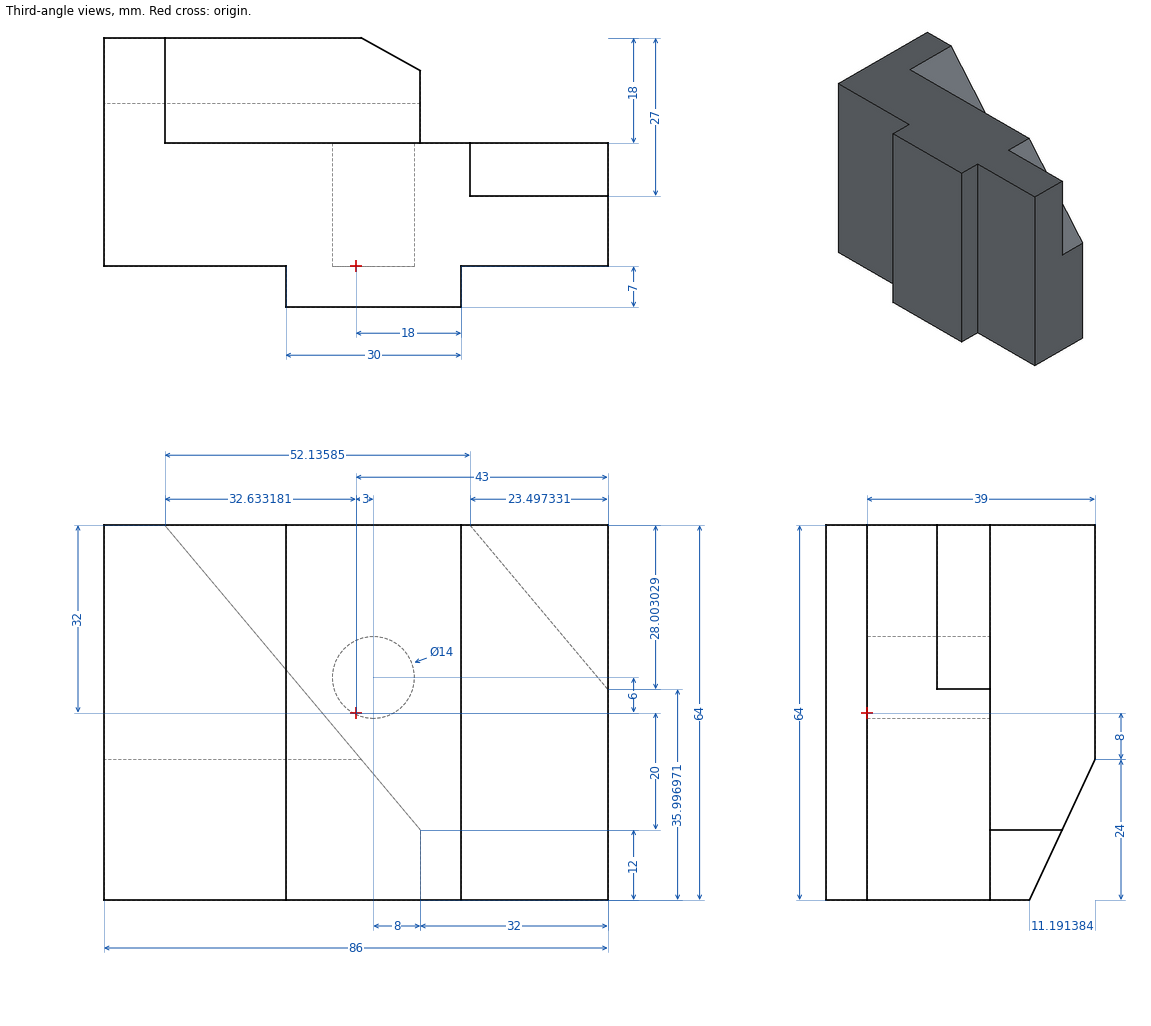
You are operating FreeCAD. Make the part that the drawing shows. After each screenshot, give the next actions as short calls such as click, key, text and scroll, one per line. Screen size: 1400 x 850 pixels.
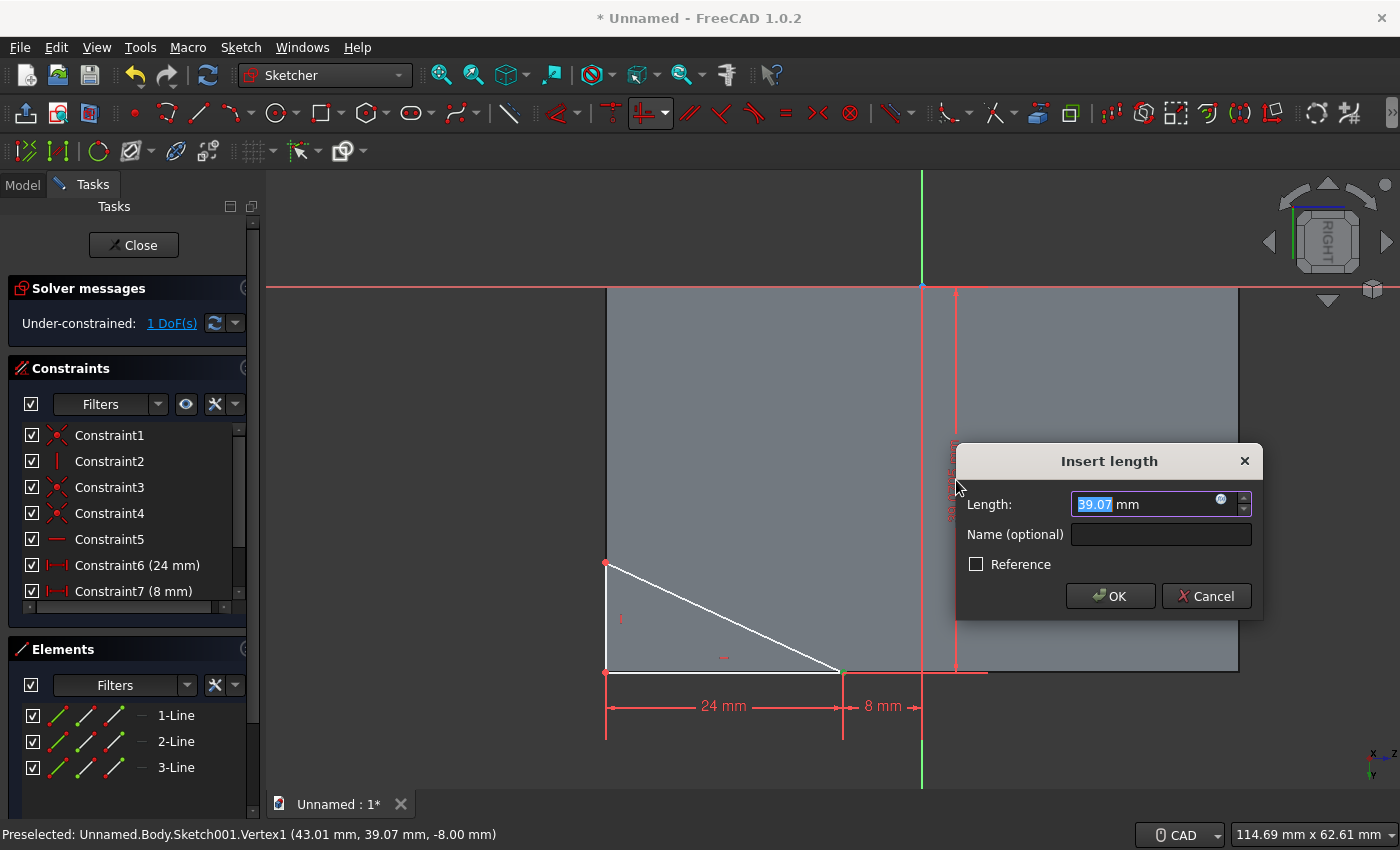
text(39)
key(Return)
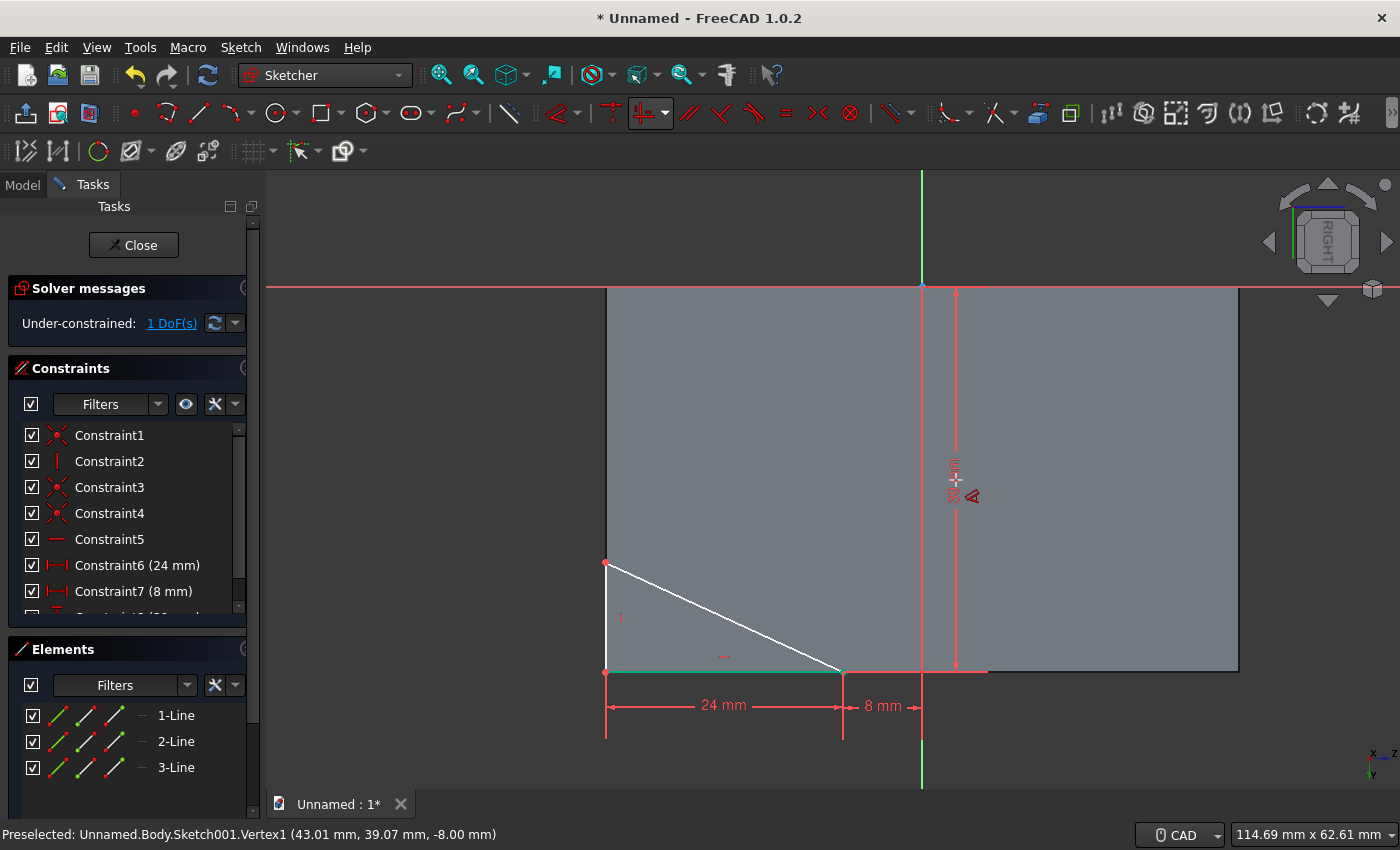
click(606, 596)
click(572, 618)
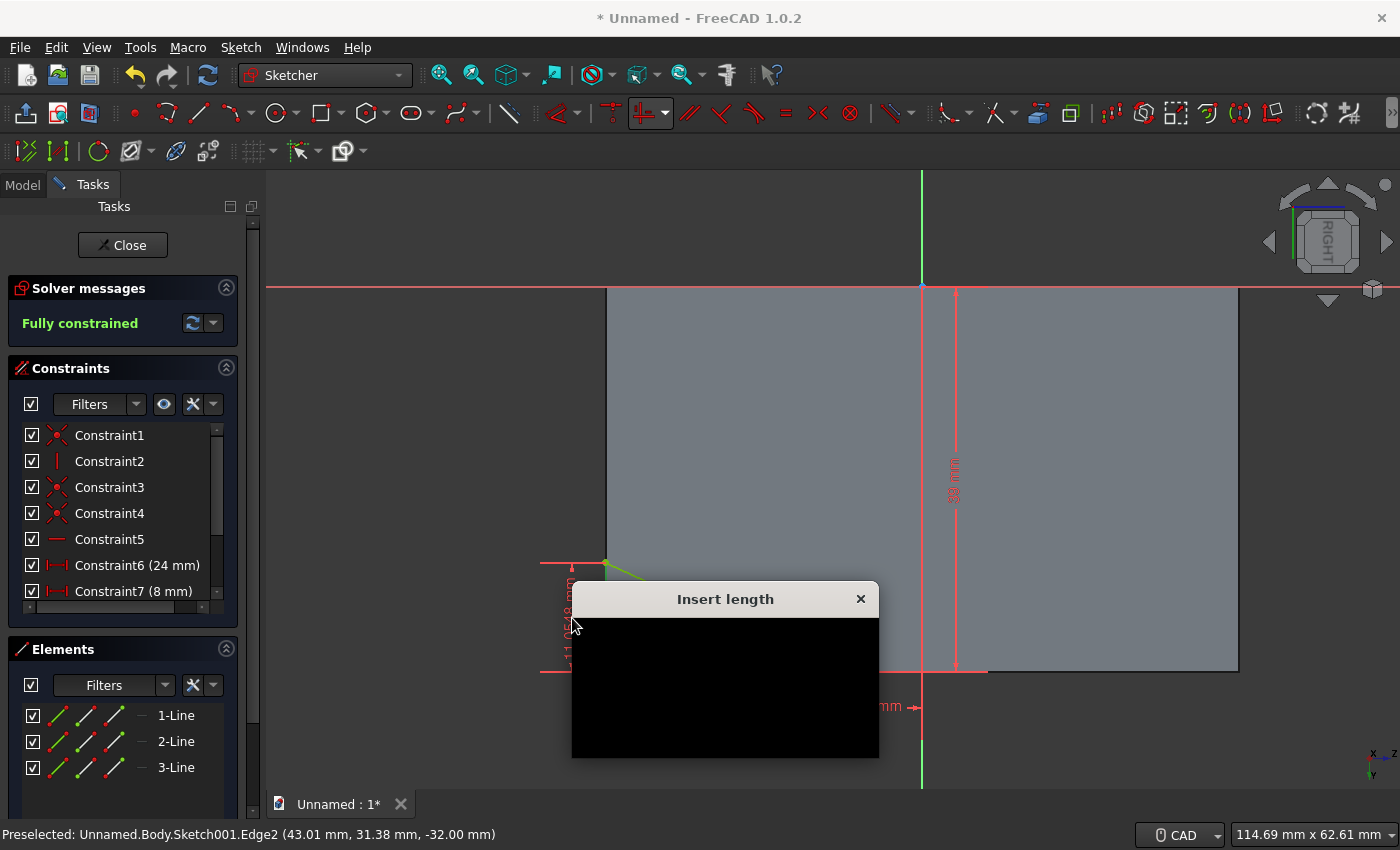
text(11.191384)
key(Return)
key(Escape)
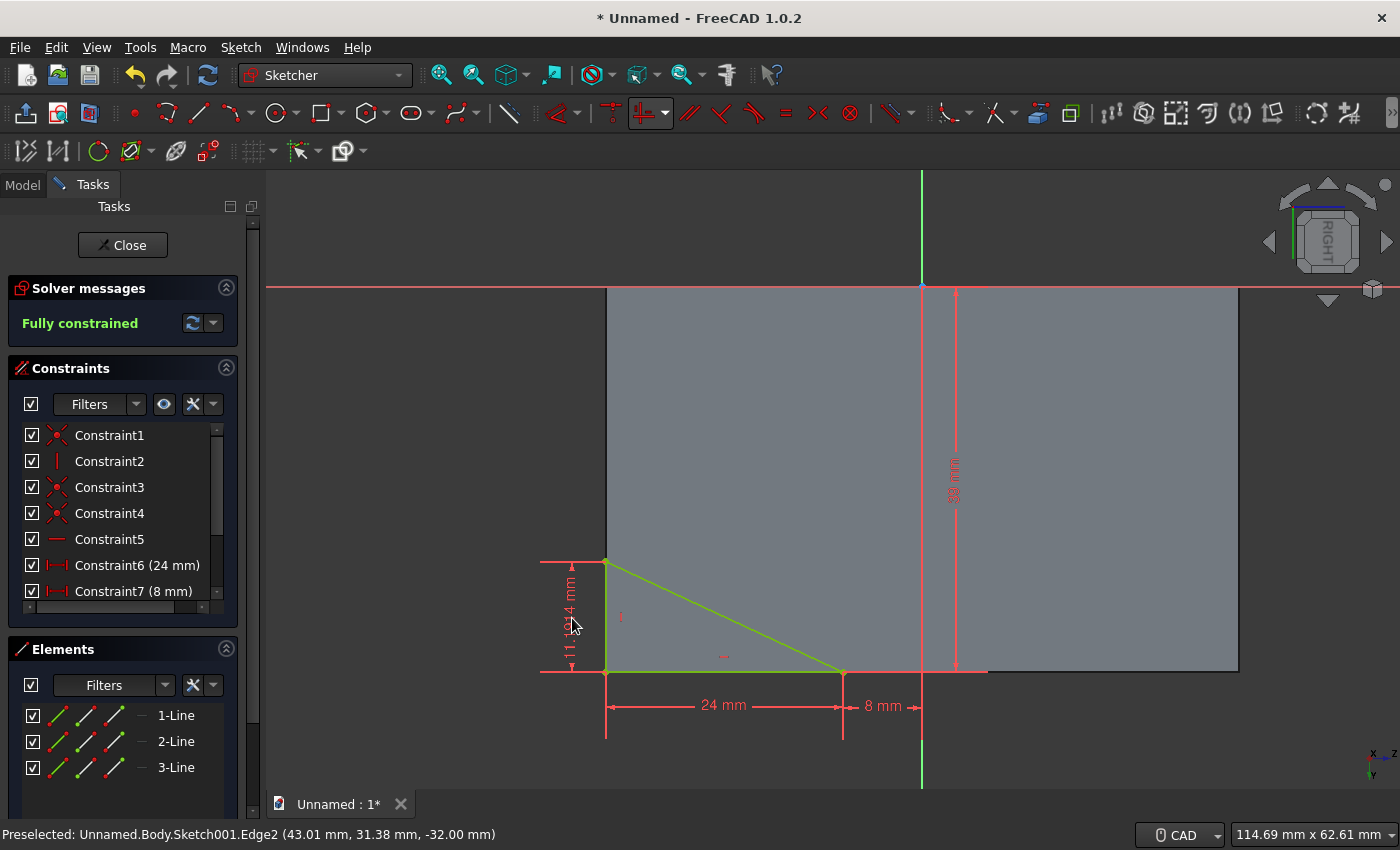
click(123, 245)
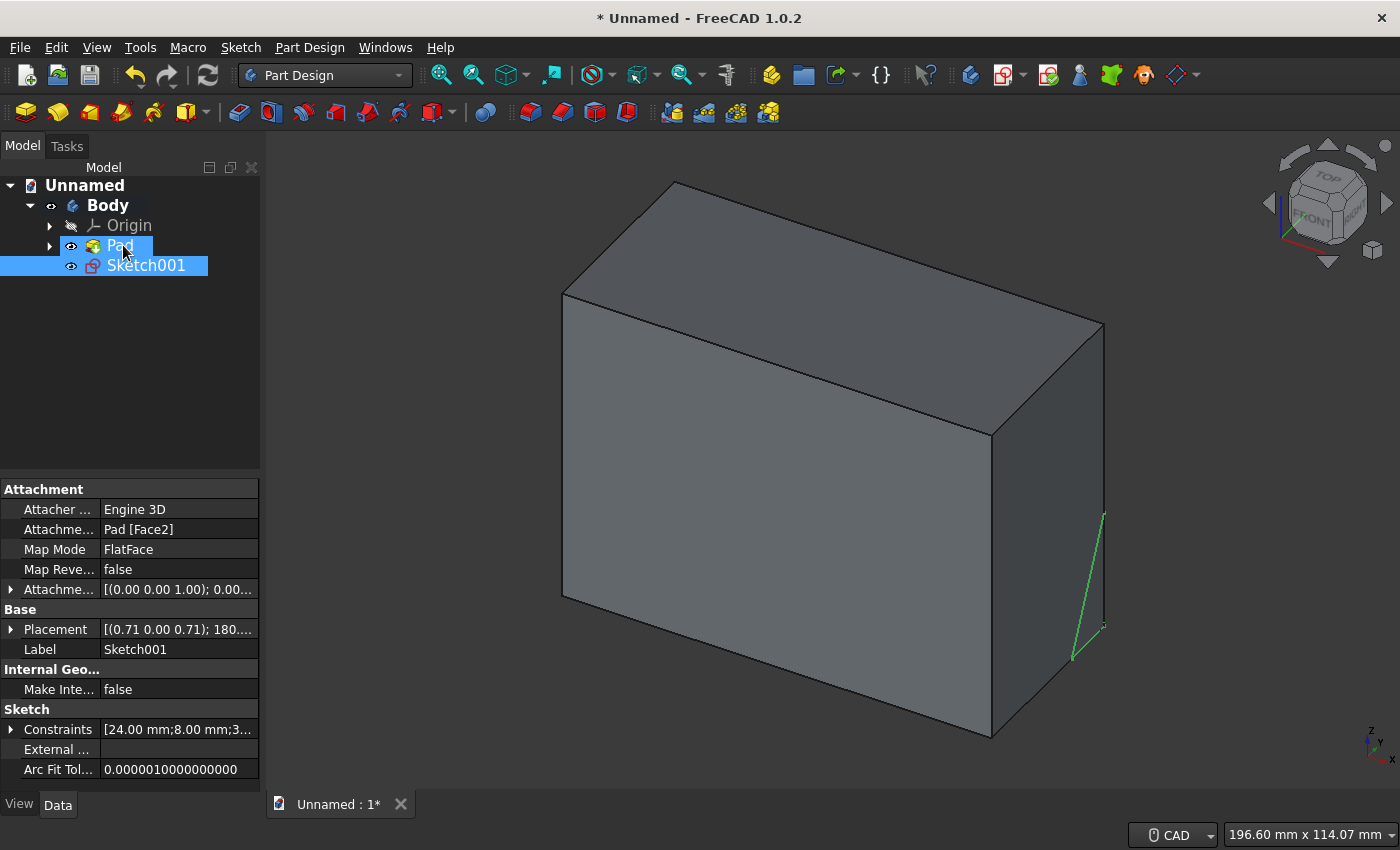
click(240, 112)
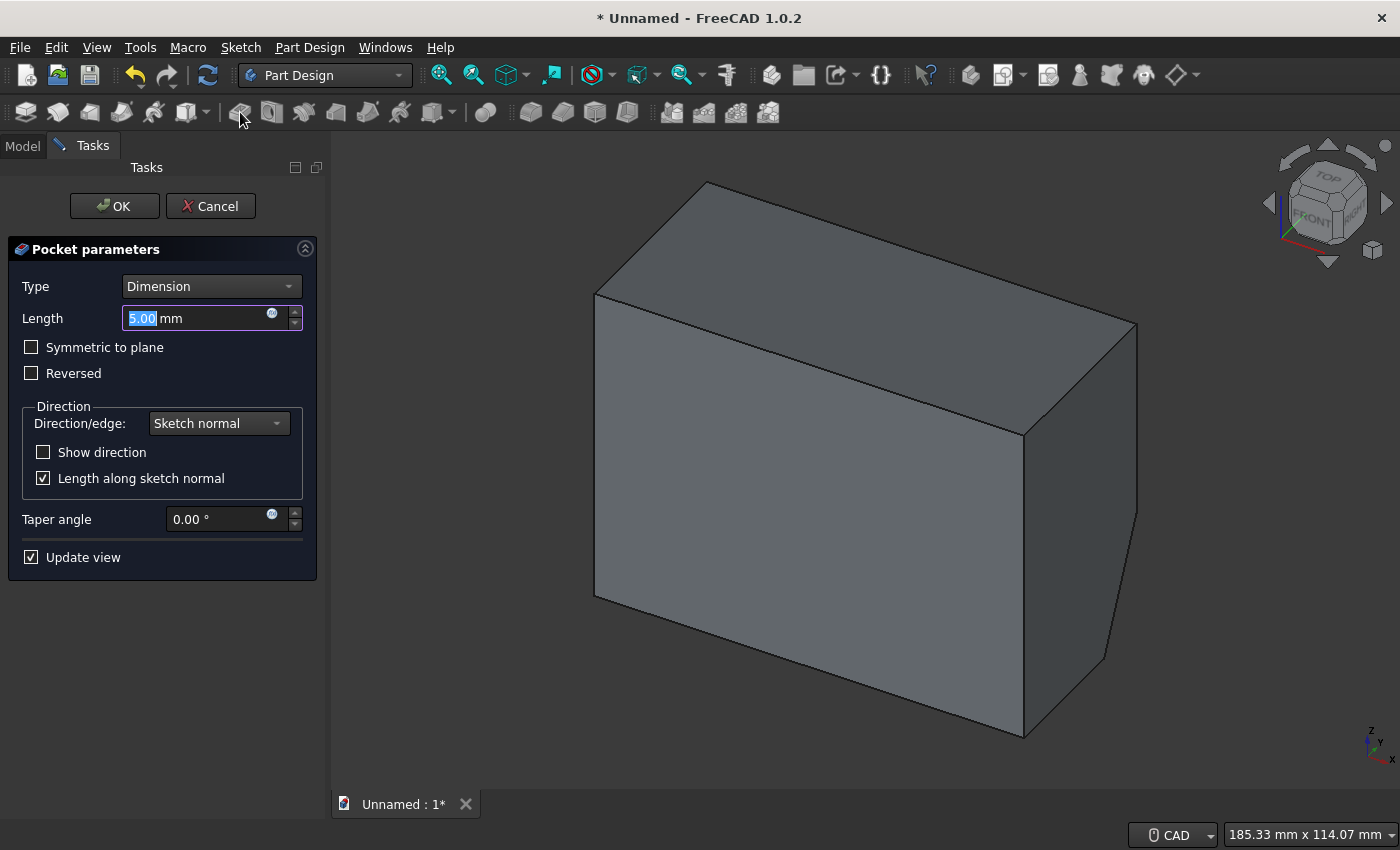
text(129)
key(Tab)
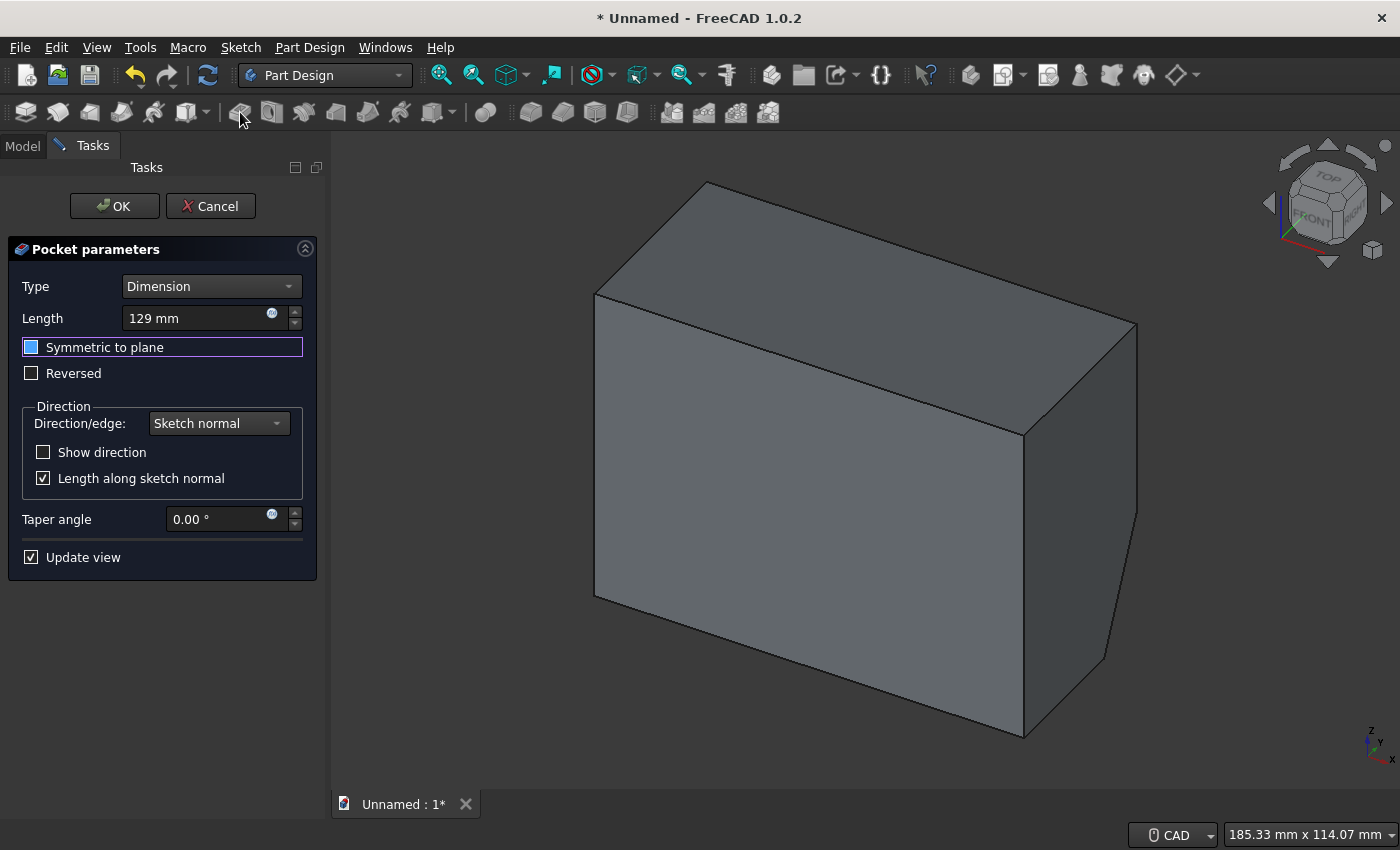
click(115, 206)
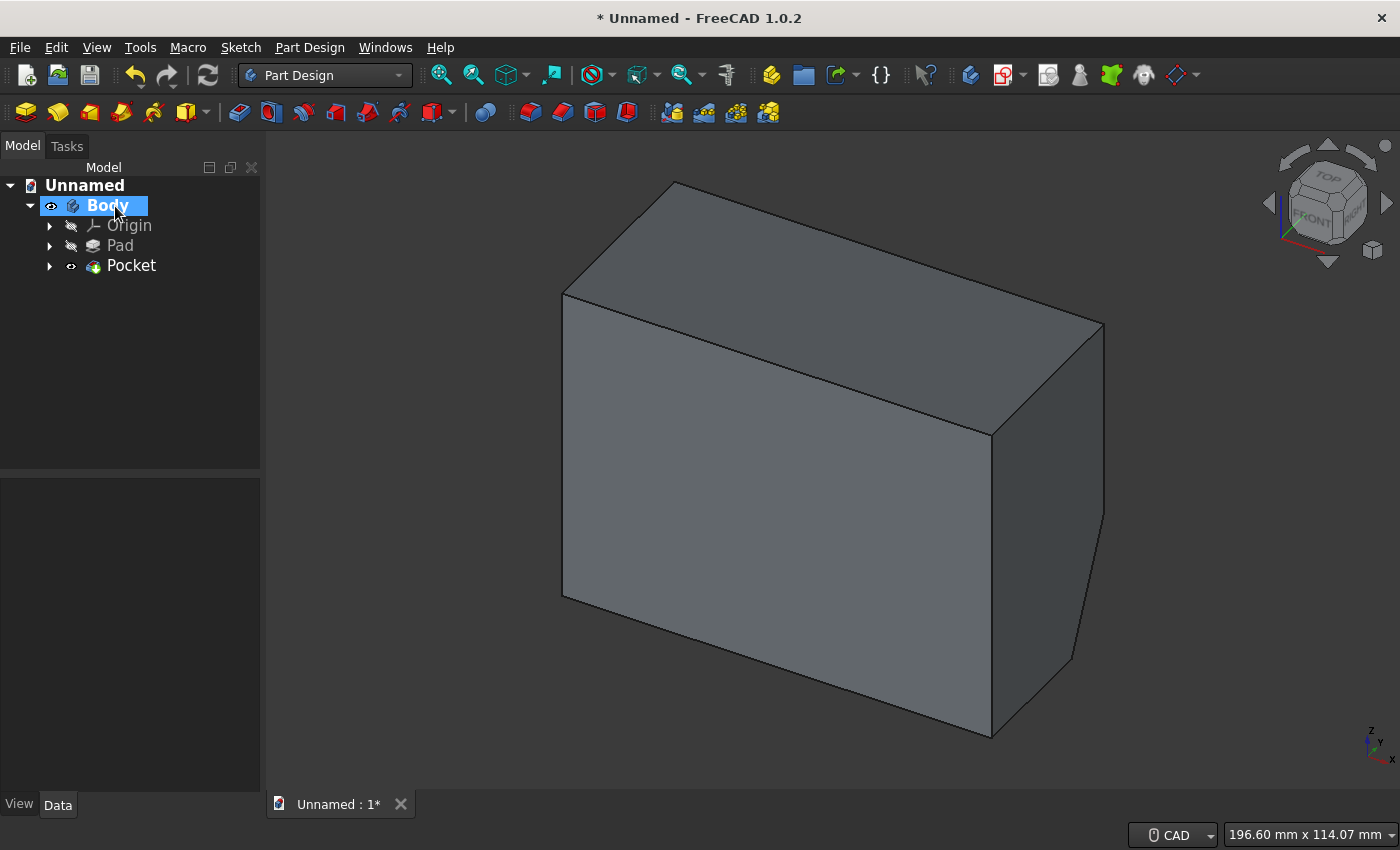
key(4)